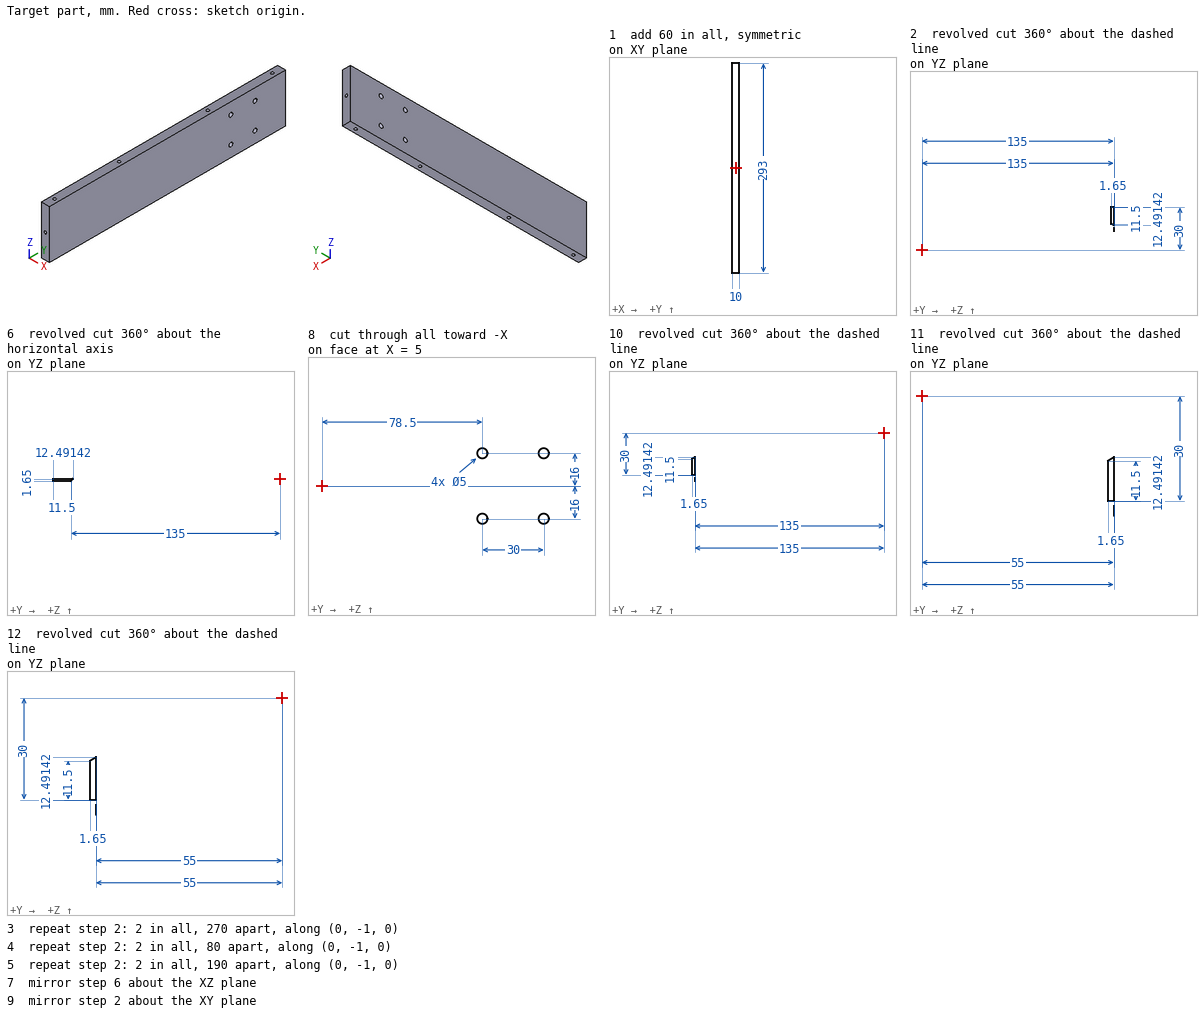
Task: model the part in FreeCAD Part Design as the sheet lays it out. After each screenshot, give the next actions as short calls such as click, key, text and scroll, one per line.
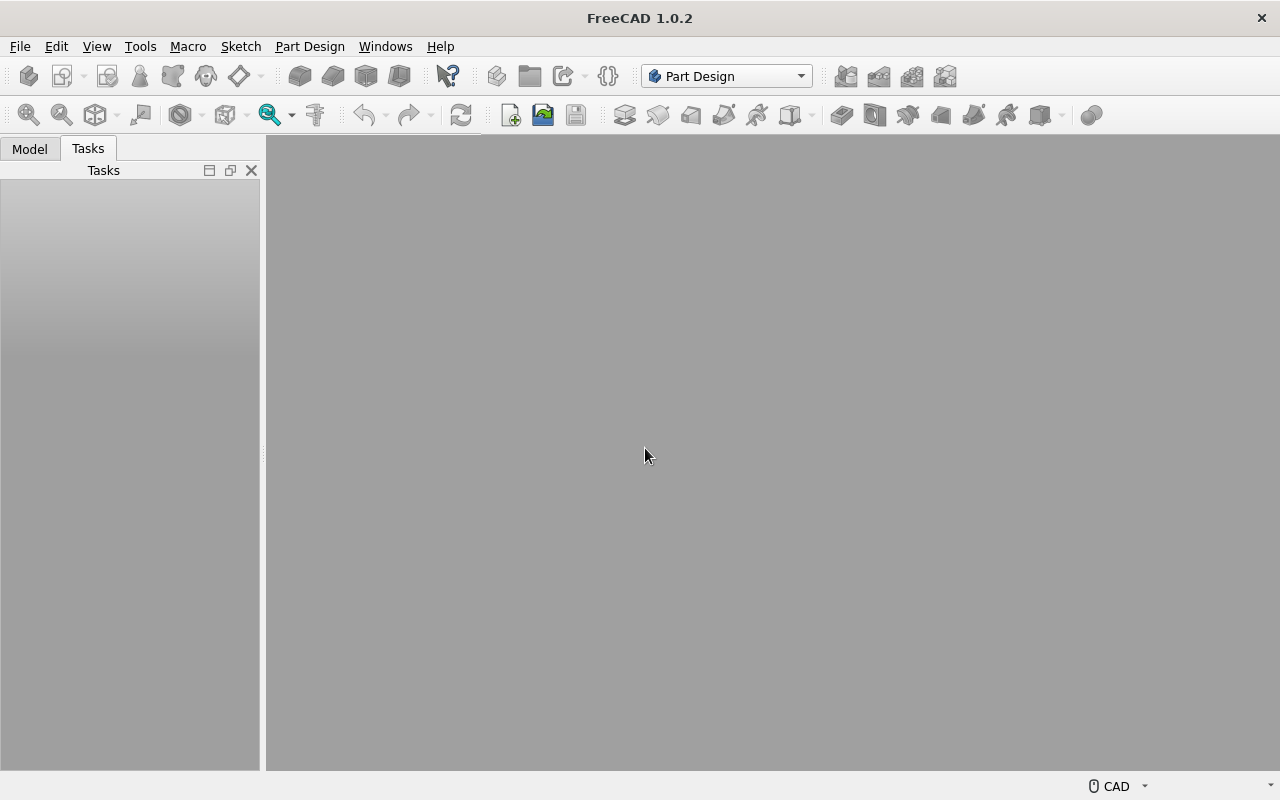
click(510, 116)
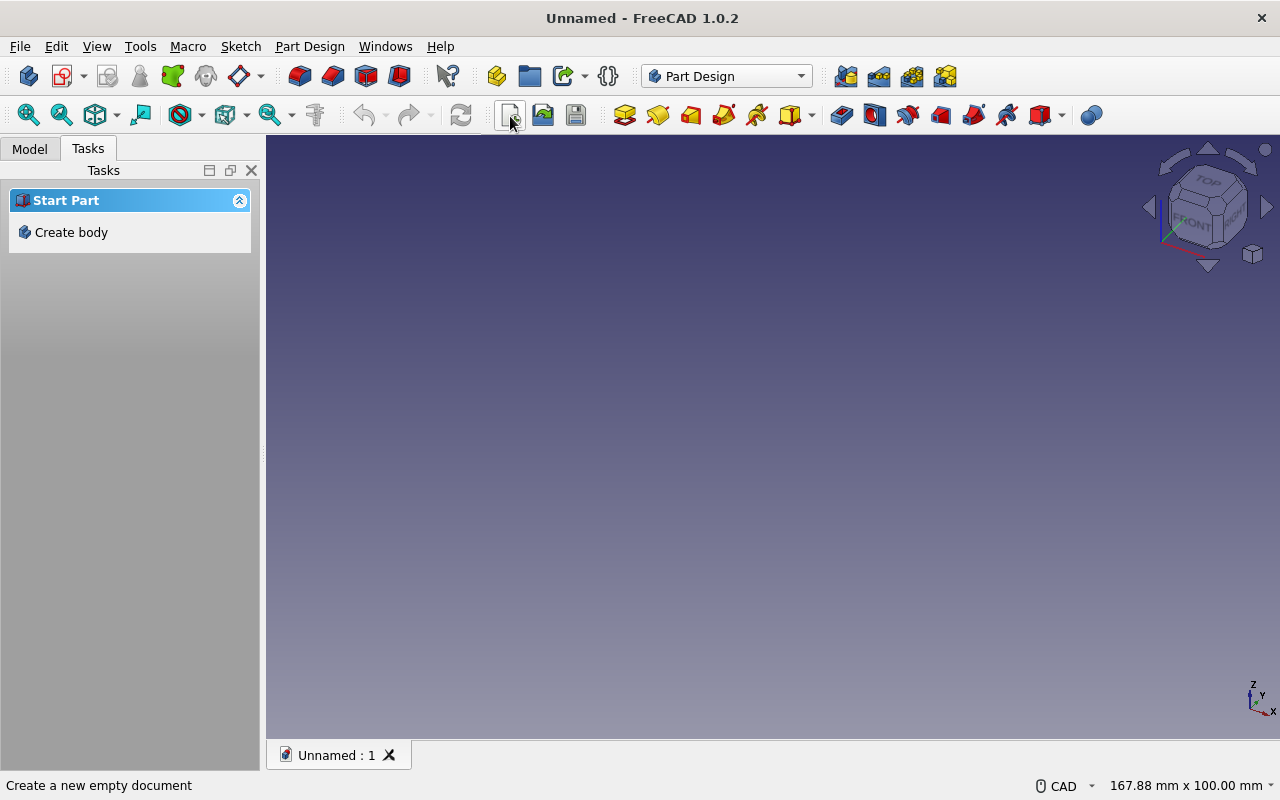
click(62, 76)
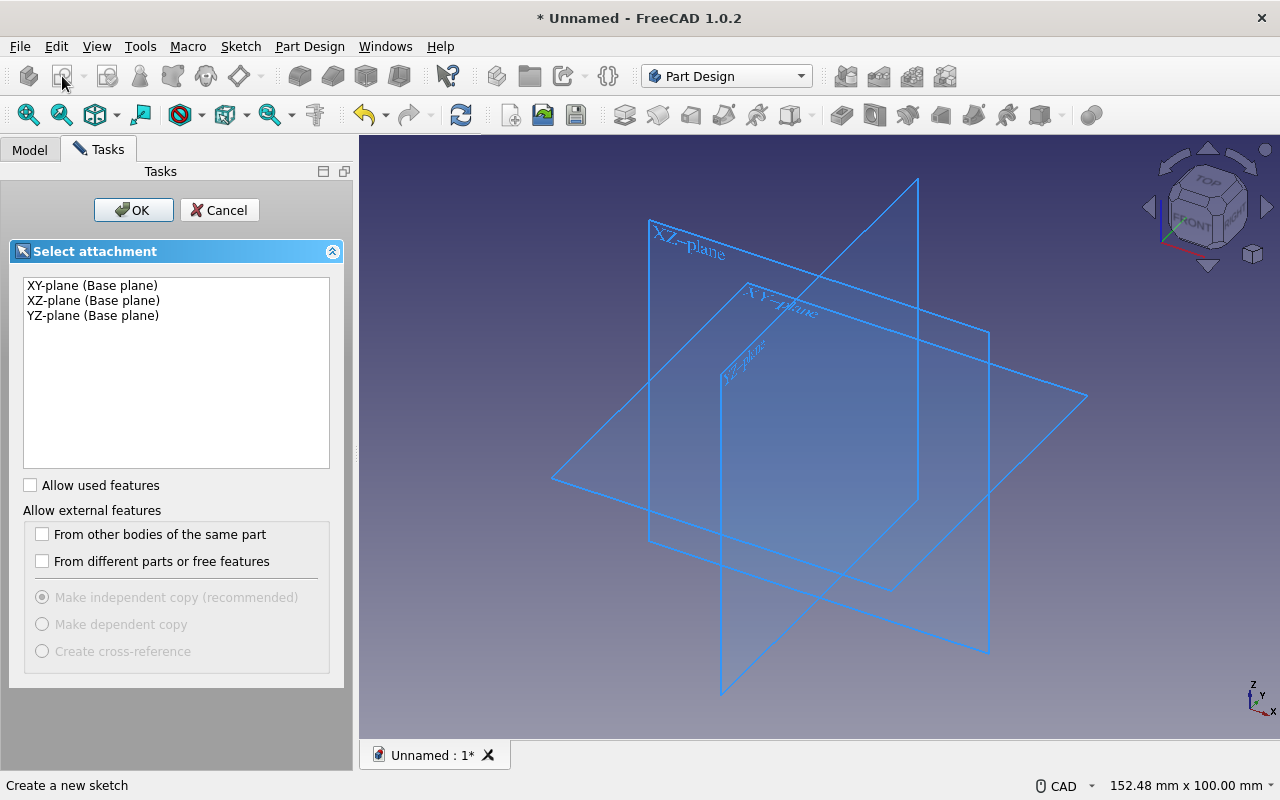
click(84, 286)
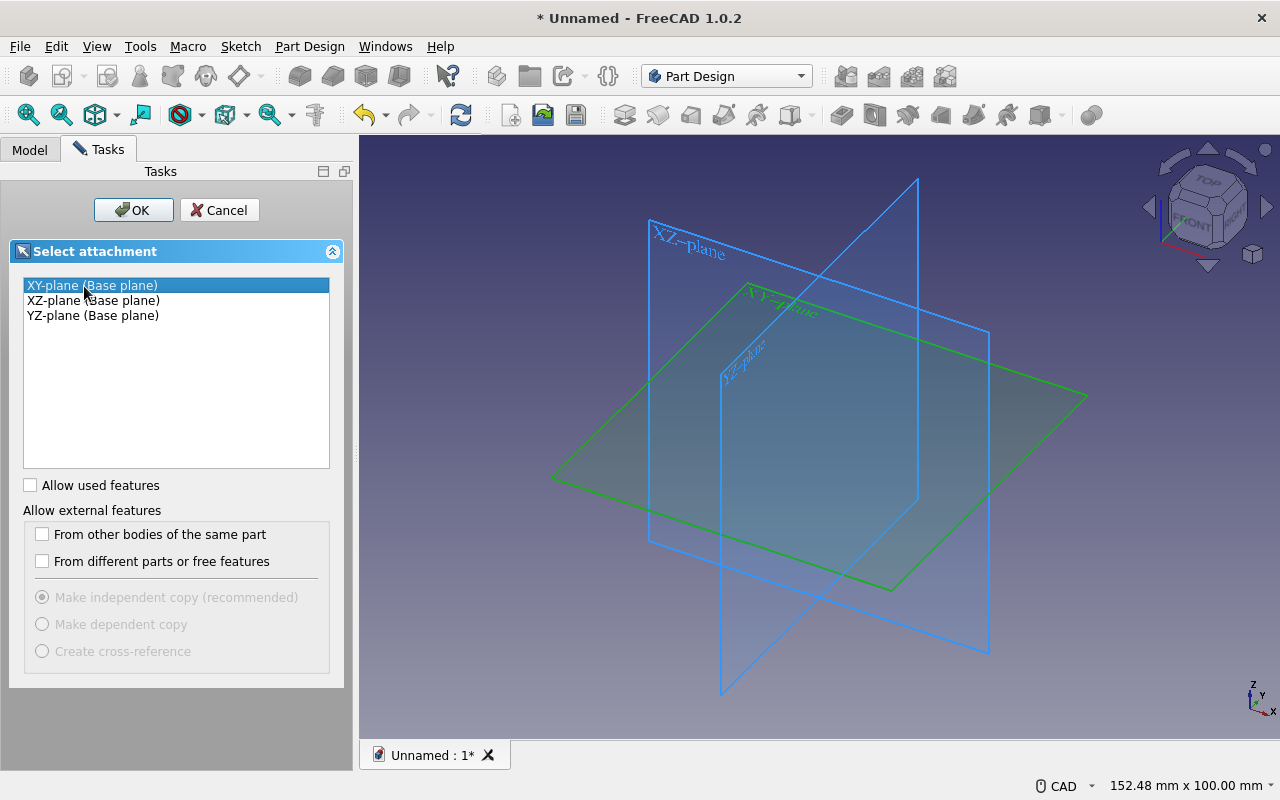
click(134, 210)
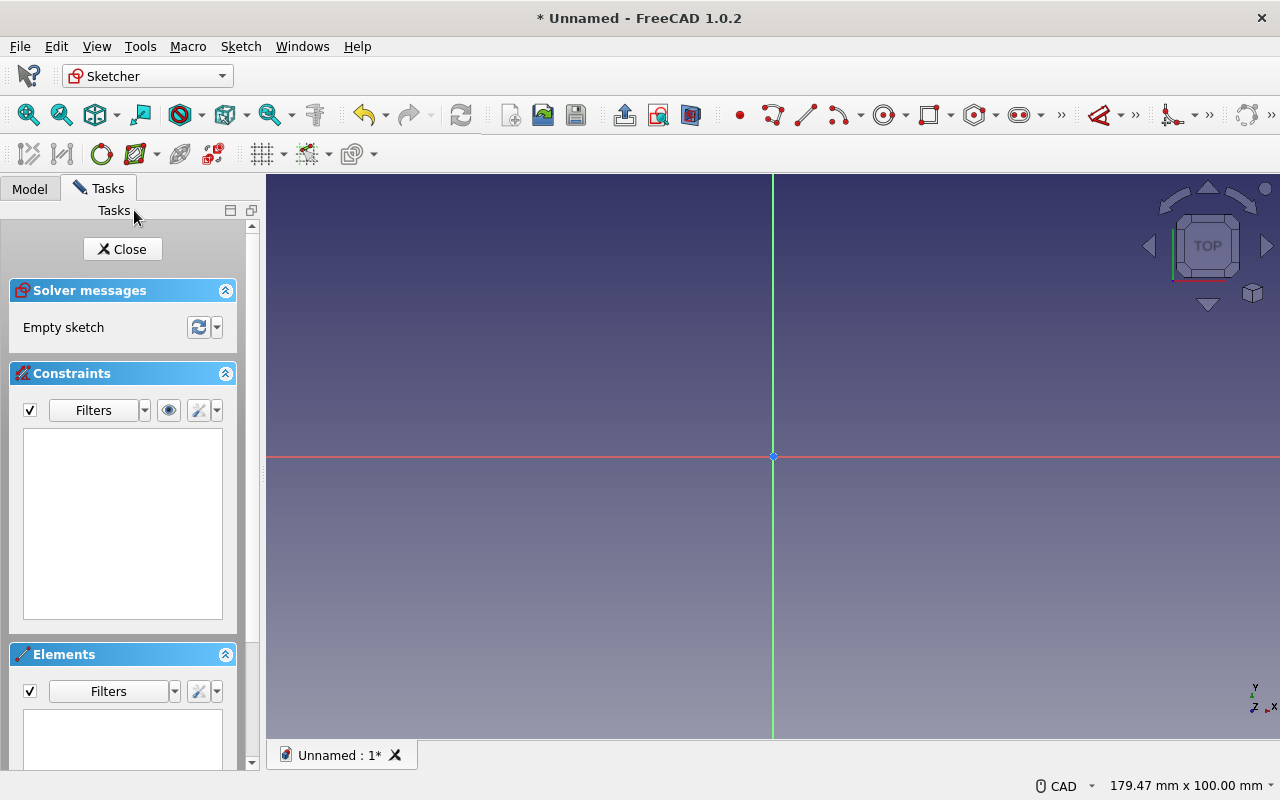
scroll(687, 456, down, 8)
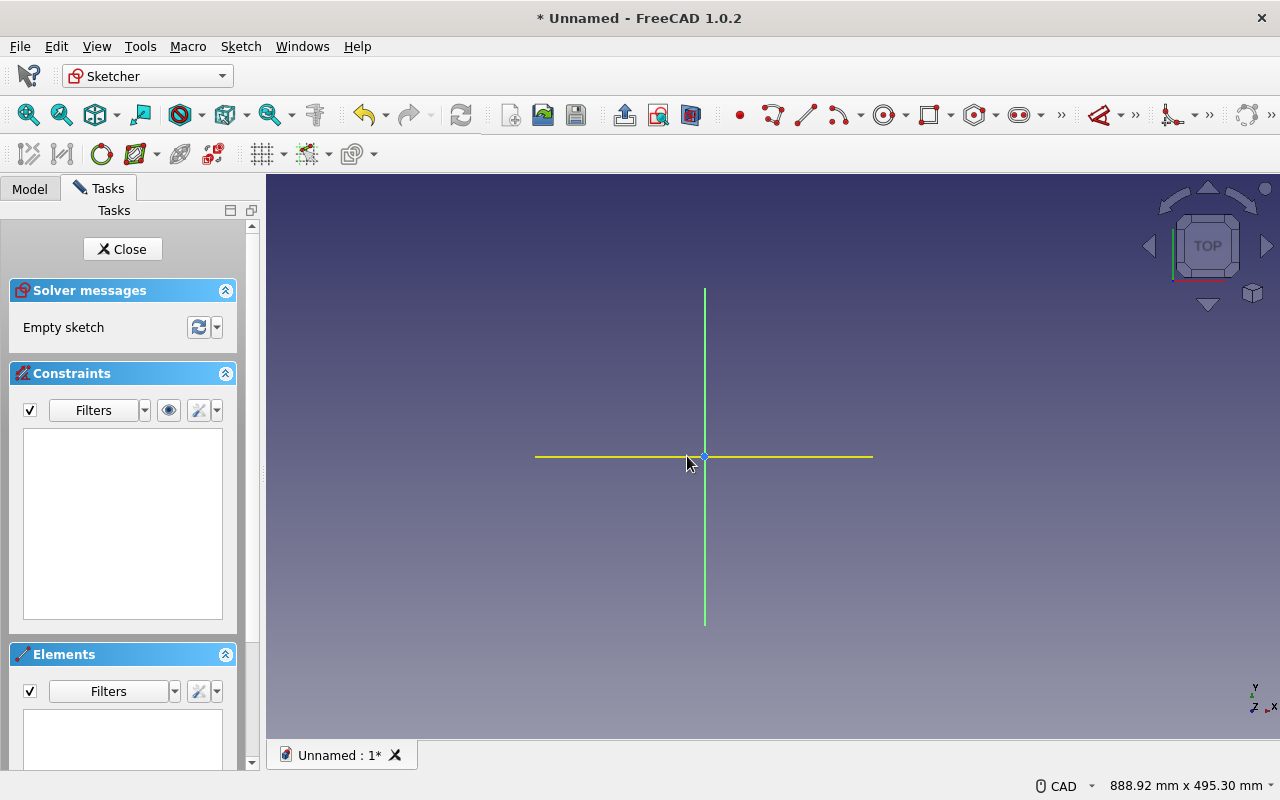
click(950, 116)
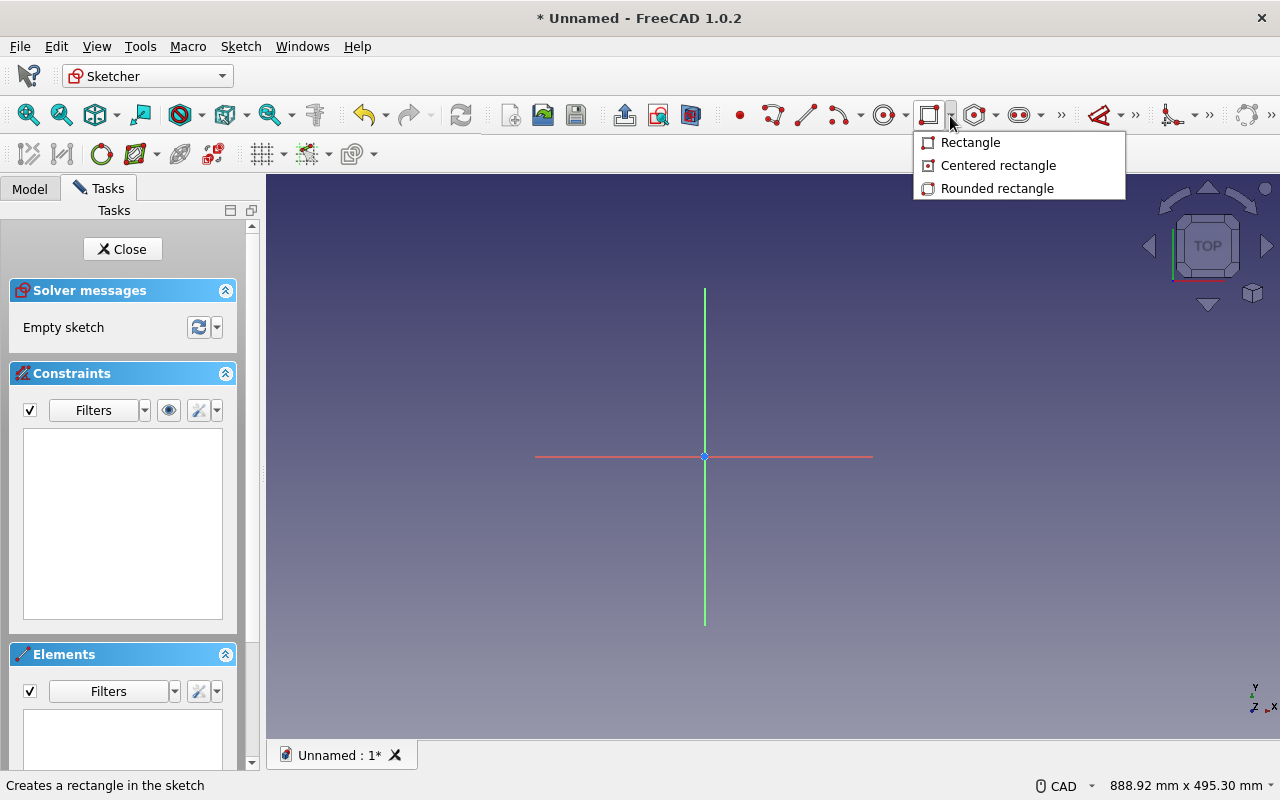
click(1020, 166)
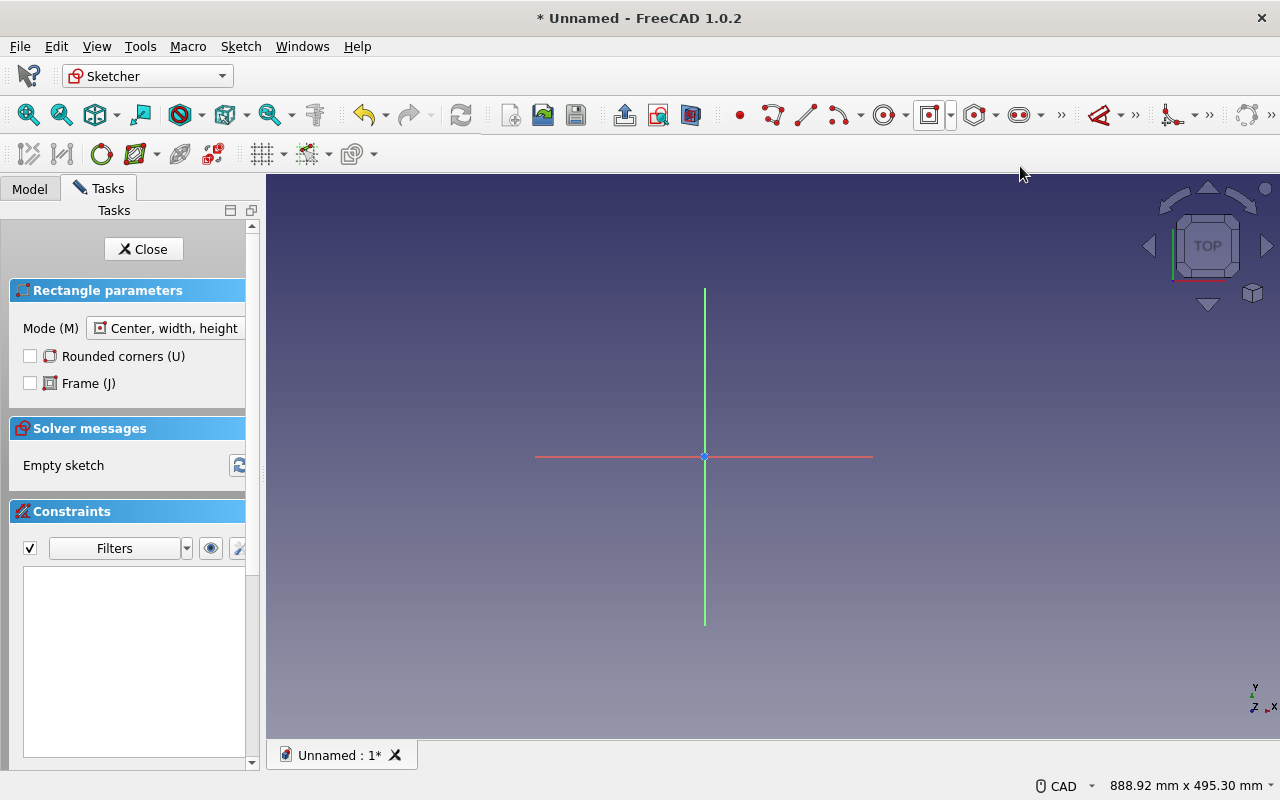
scroll(705, 456, up, 6)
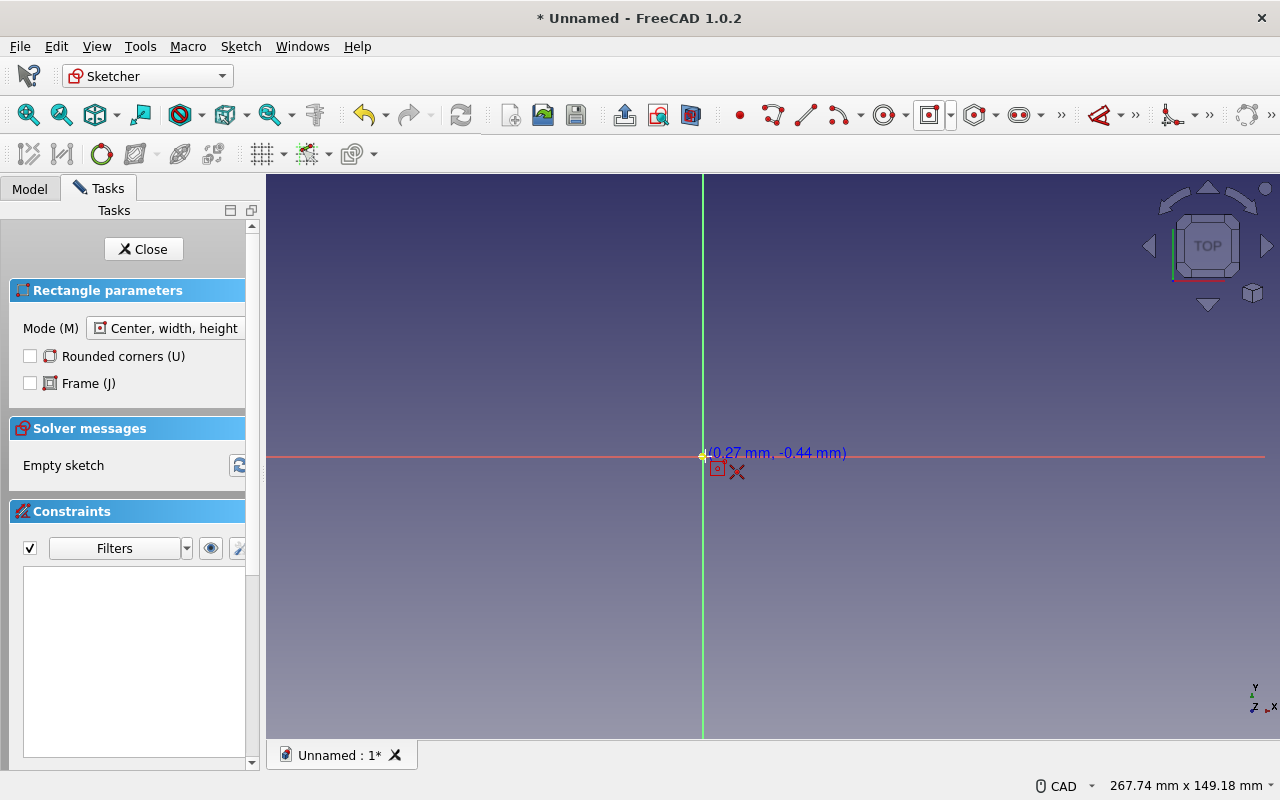
click(703, 456)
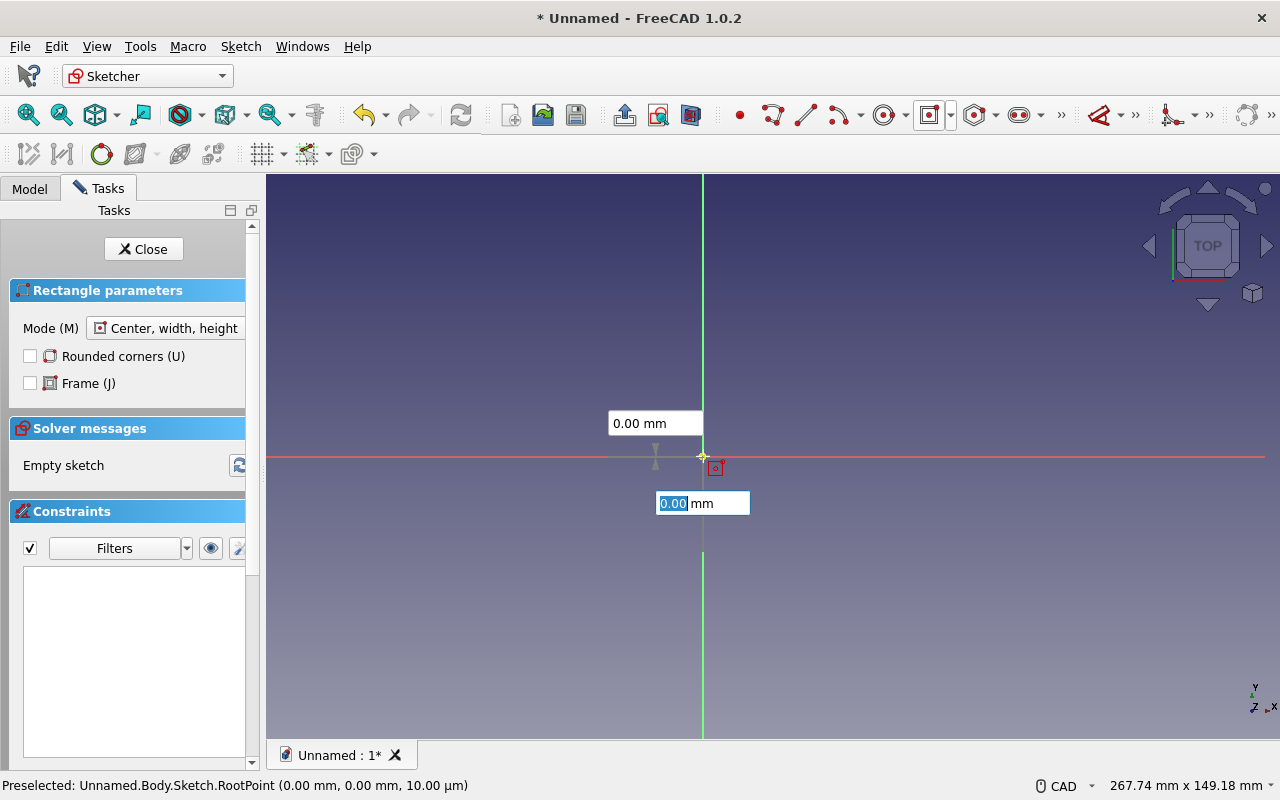
scroll(705, 456, down, 6)